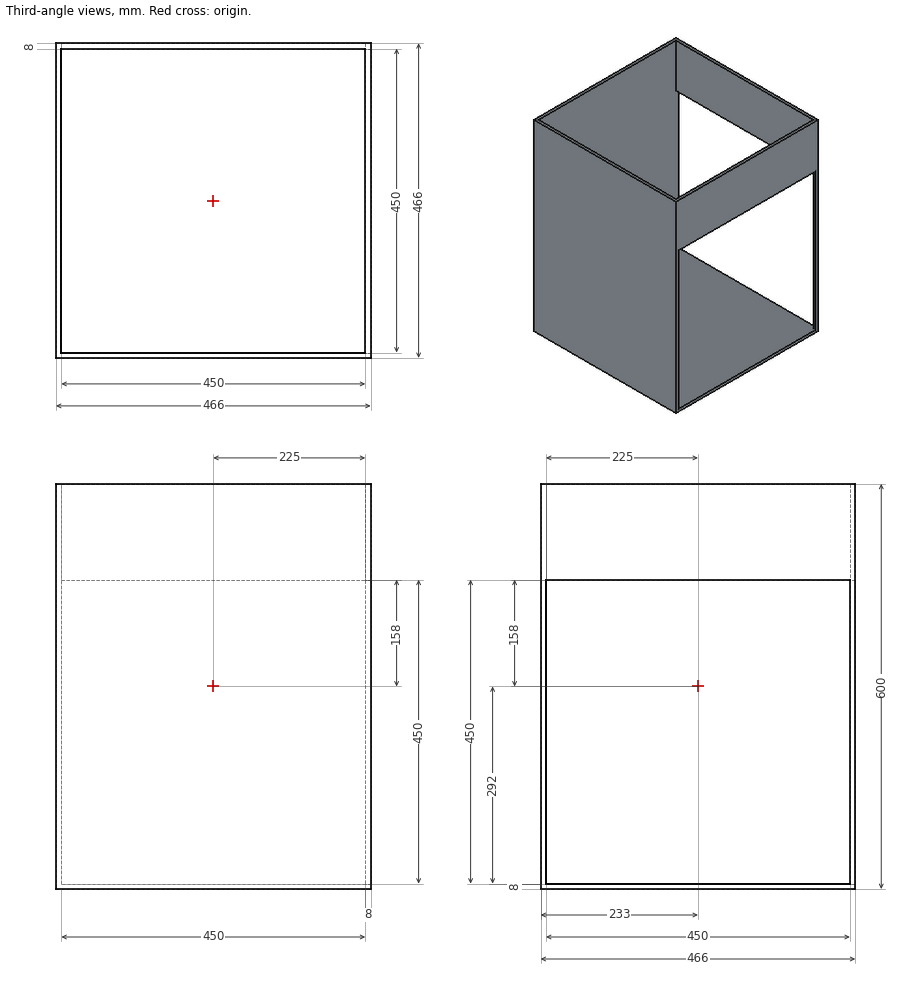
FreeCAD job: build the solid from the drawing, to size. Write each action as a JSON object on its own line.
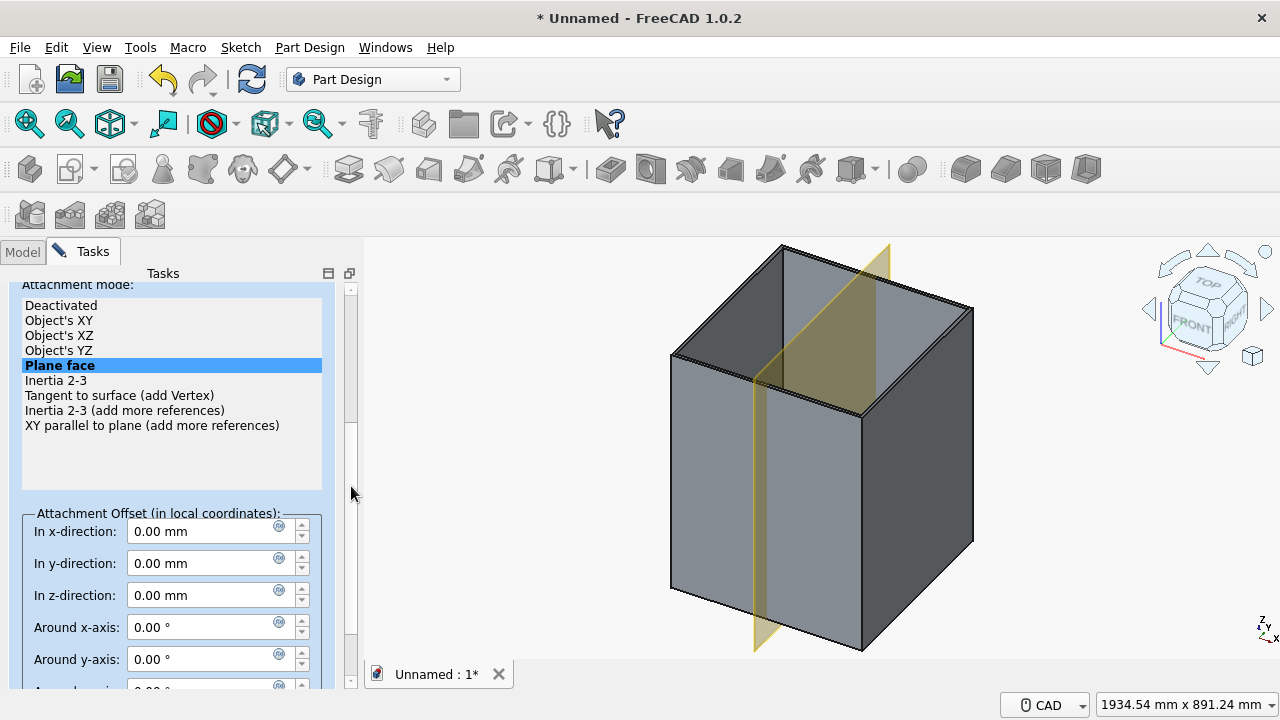
{"action": "triple_click", "coordinate": [210, 595]}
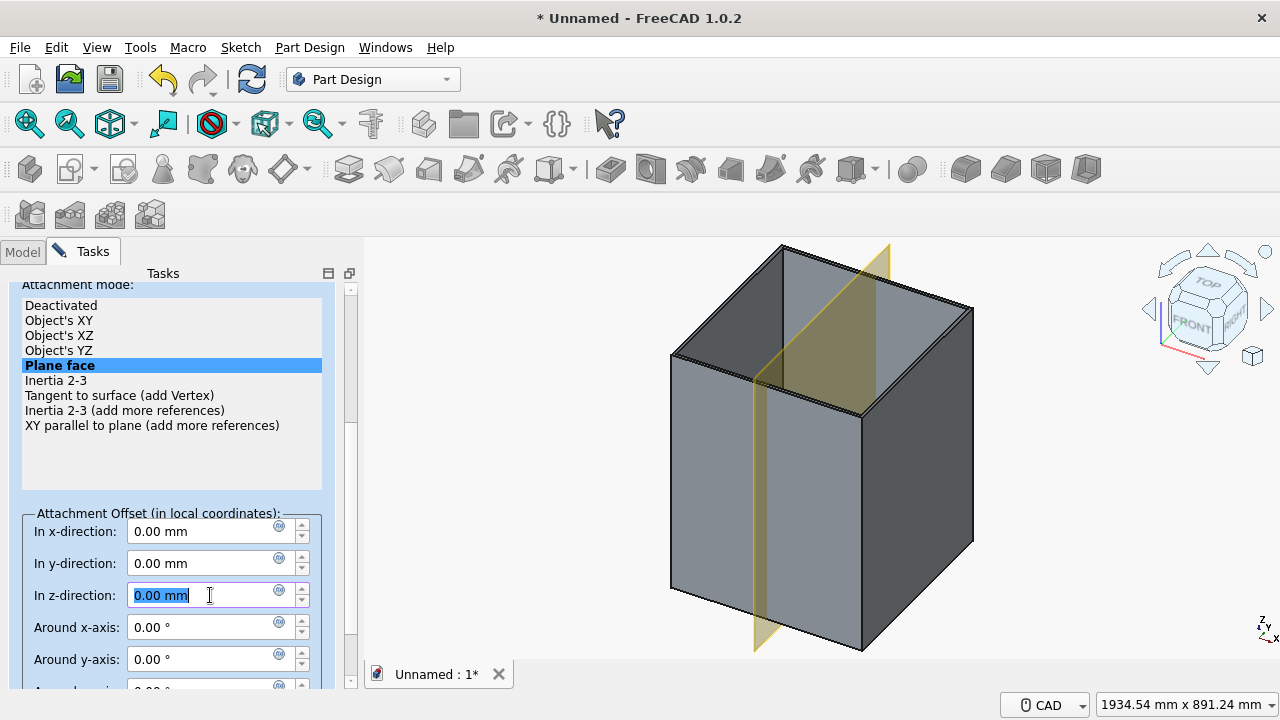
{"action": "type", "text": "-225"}
{"action": "key", "text": "Tab"}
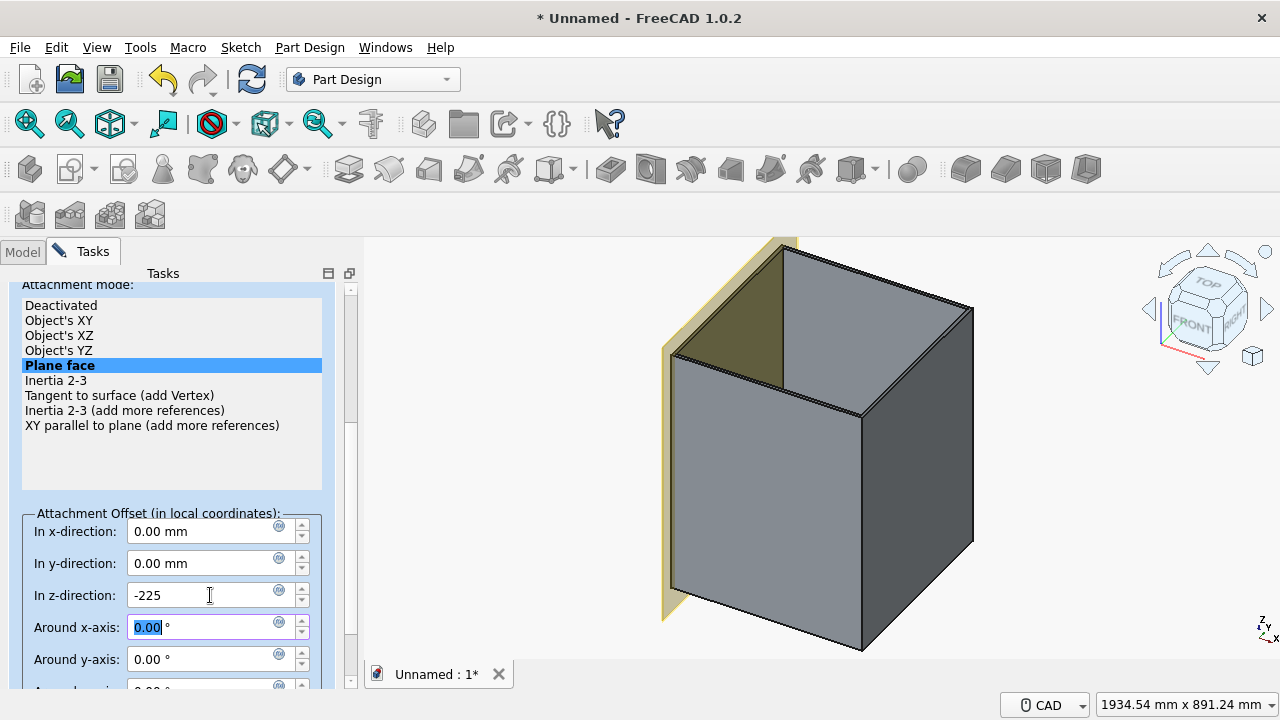
{"action": "scroll", "coordinate": [351, 486], "scroll_direction": "up", "scroll_amount": 5}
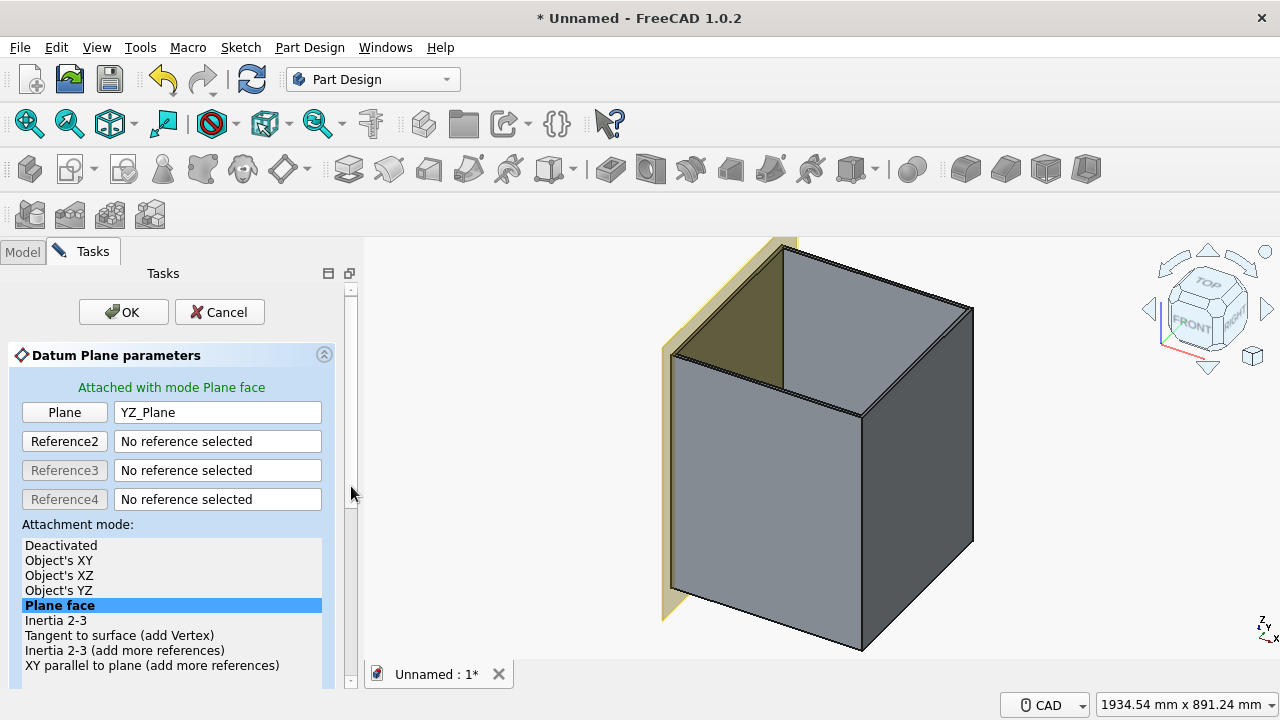
{"action": "left_click", "coordinate": [124, 312]}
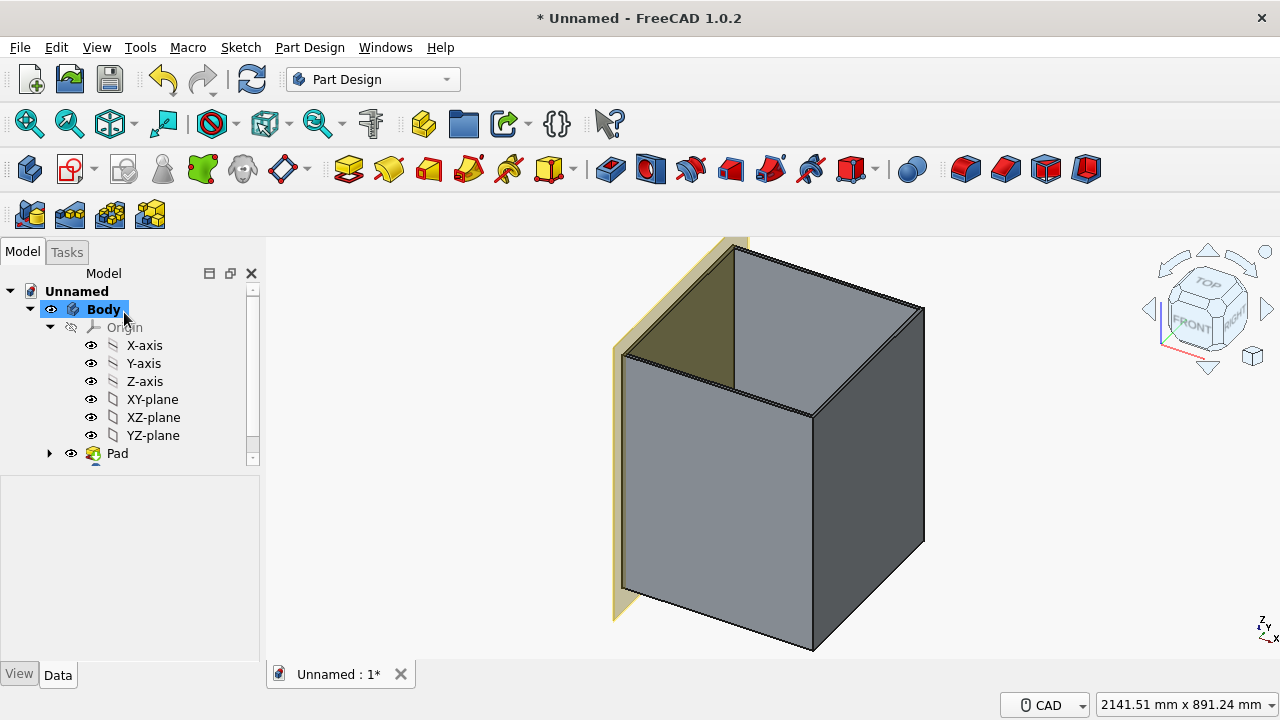
{"action": "scroll", "coordinate": [100, 377], "scroll_direction": "down", "scroll_amount": 3}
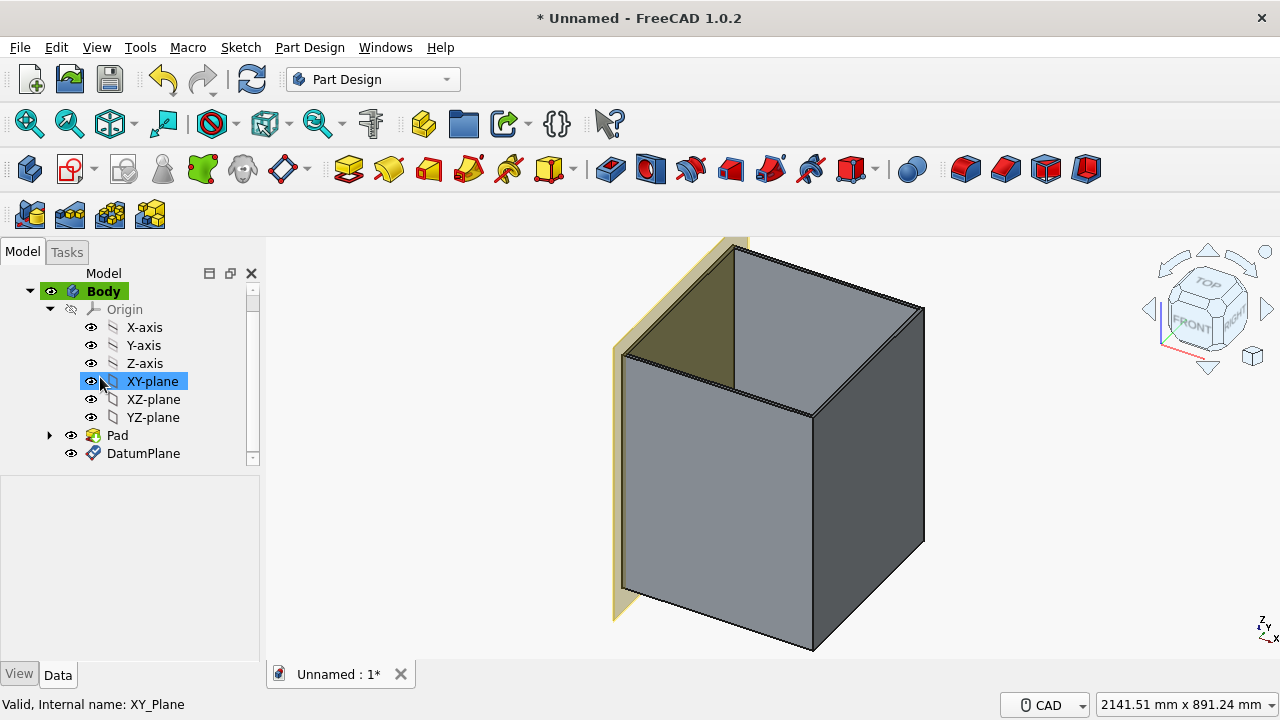
{"action": "left_click", "coordinate": [116, 453]}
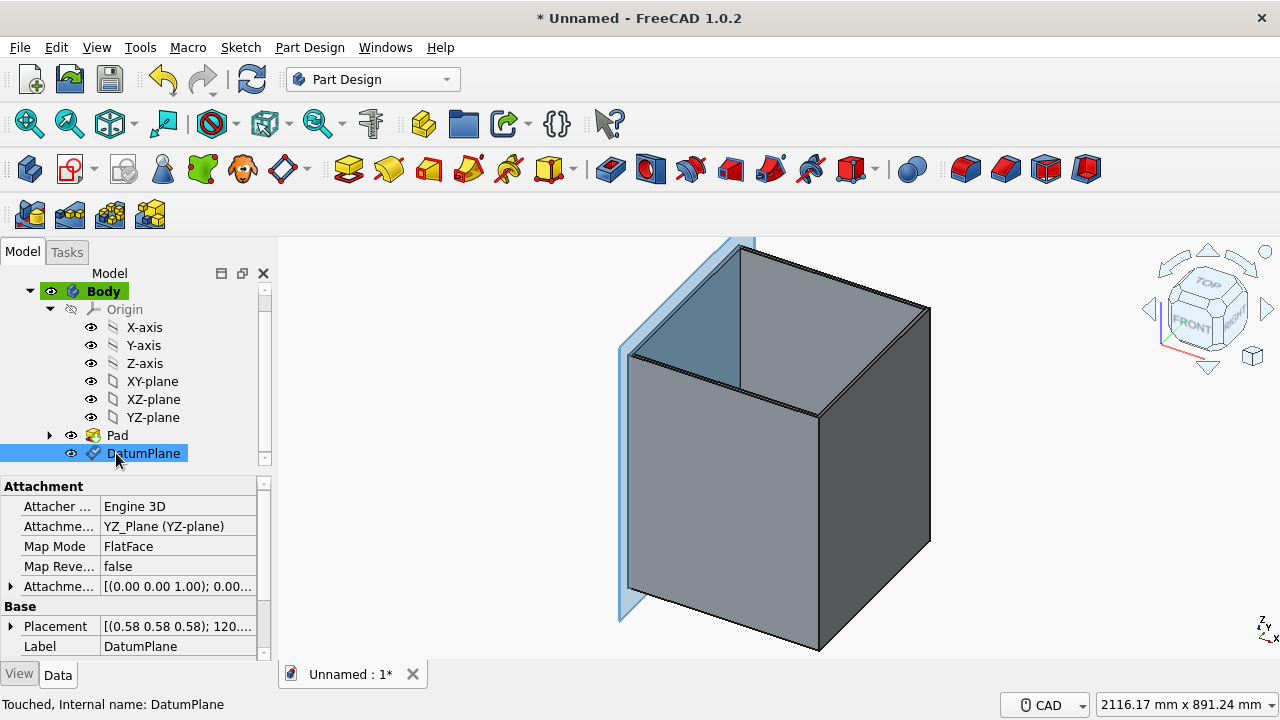
{"action": "left_click", "coordinate": [70, 170]}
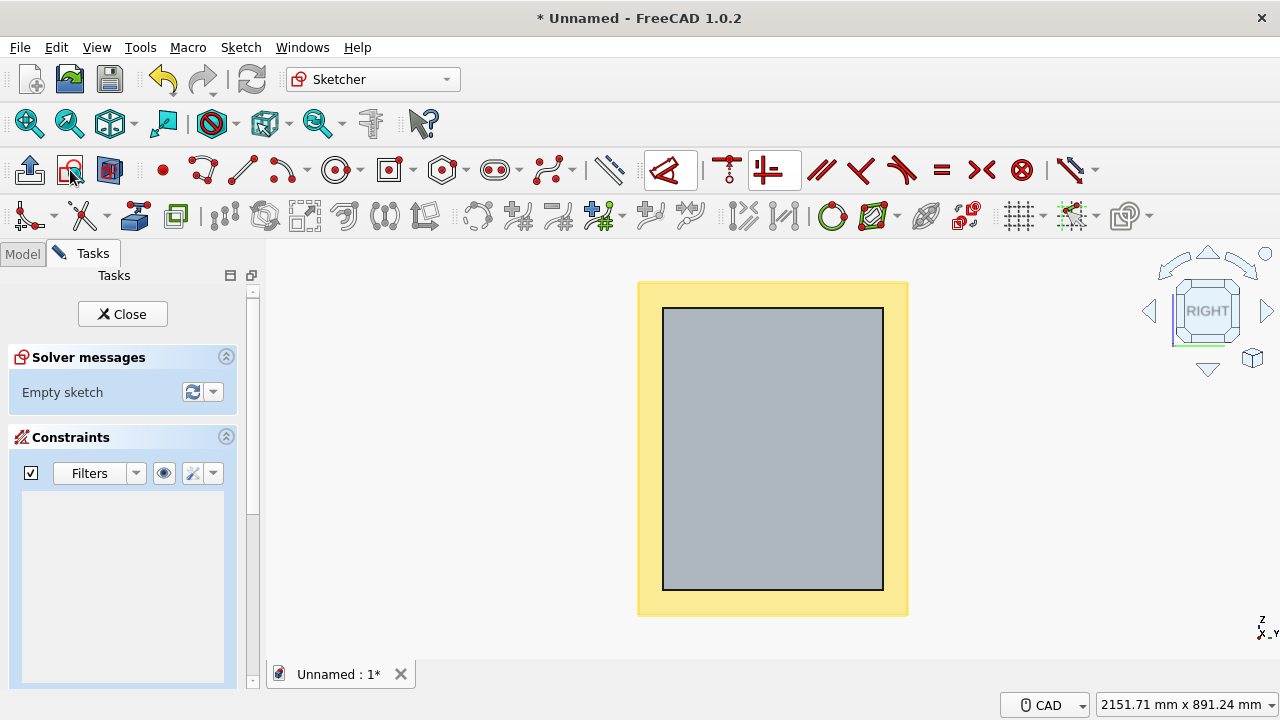
{"action": "left_click", "coordinate": [110, 170]}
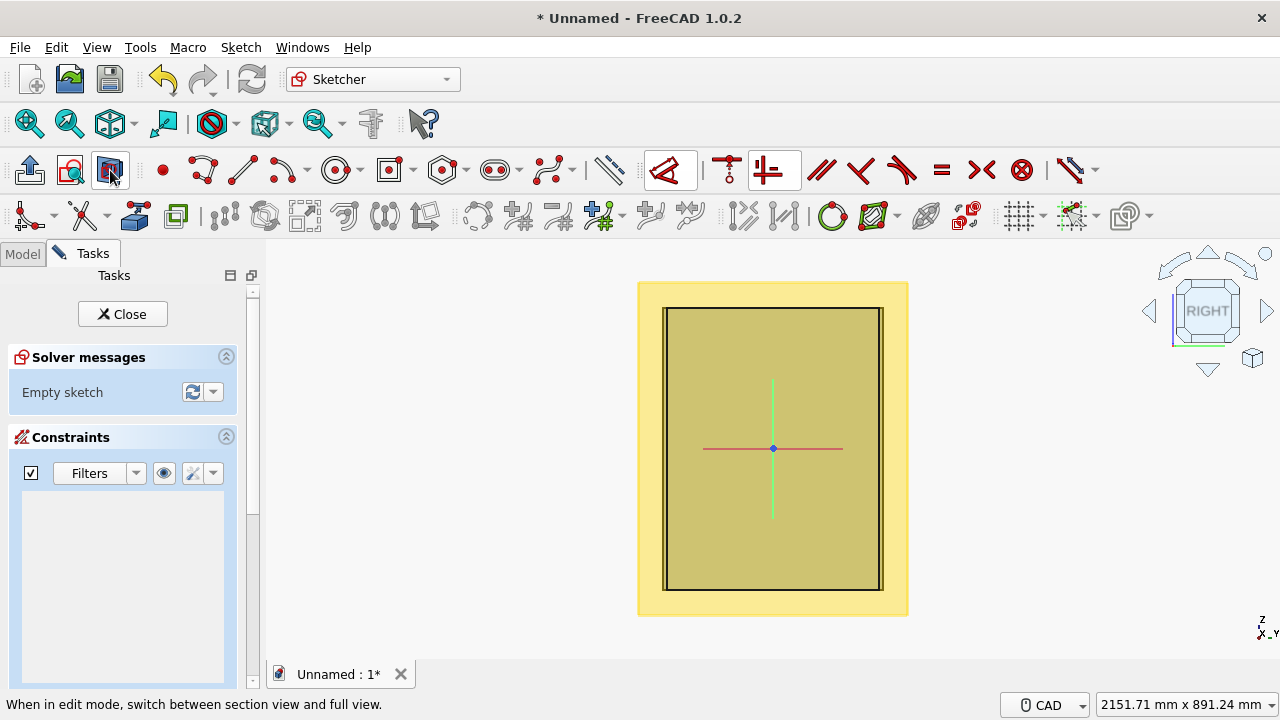
{"action": "scroll", "coordinate": [856, 606], "scroll_direction": "up", "scroll_amount": 3}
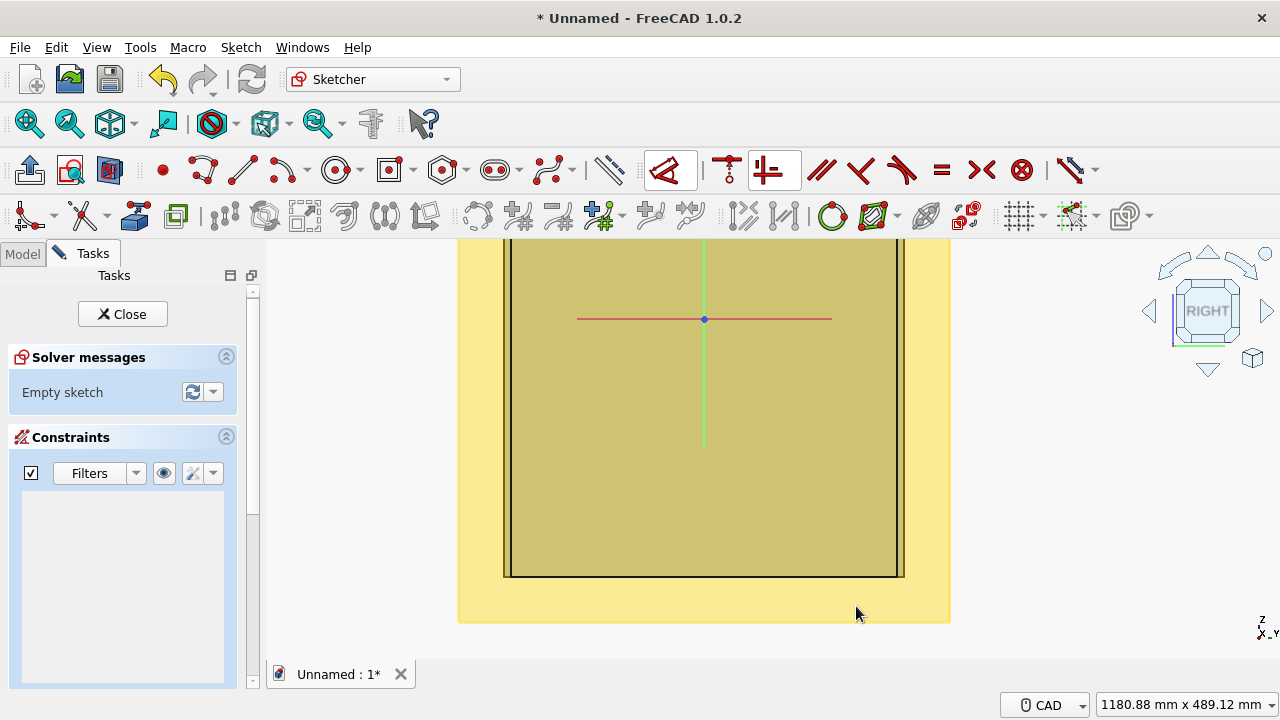
{"action": "left_click", "coordinate": [416, 170]}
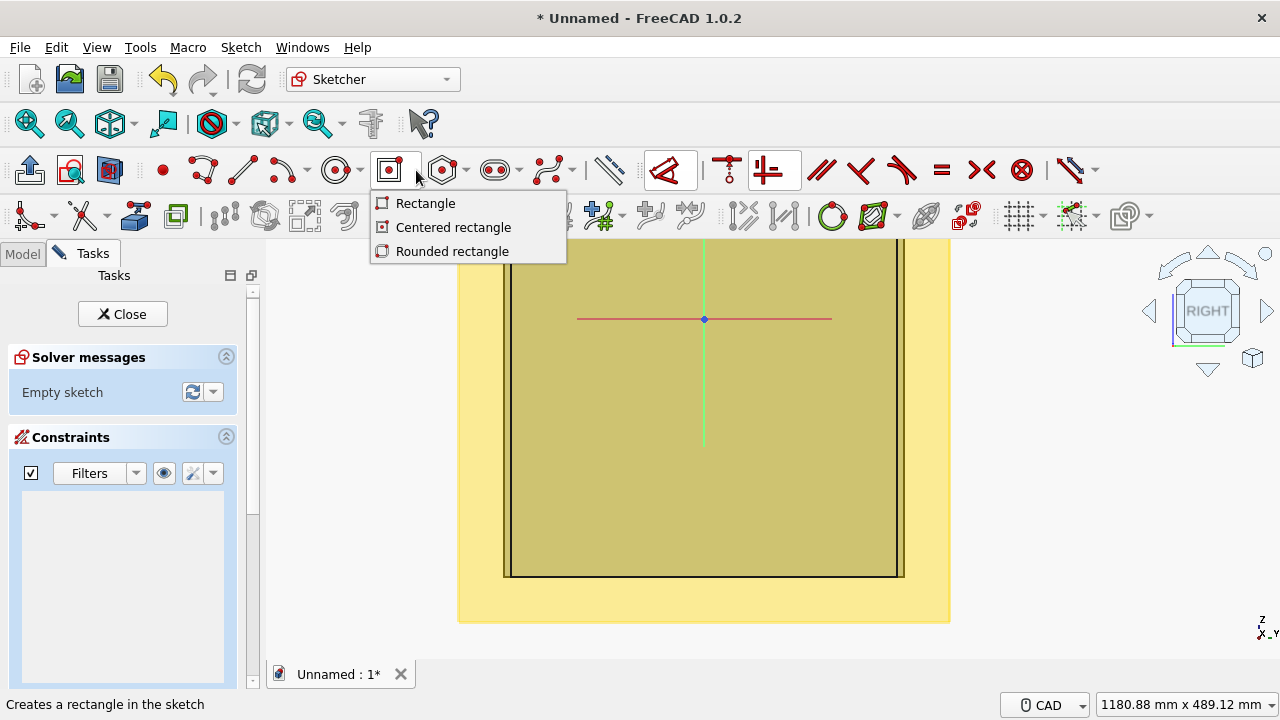
{"action": "left_click", "coordinate": [468, 203]}